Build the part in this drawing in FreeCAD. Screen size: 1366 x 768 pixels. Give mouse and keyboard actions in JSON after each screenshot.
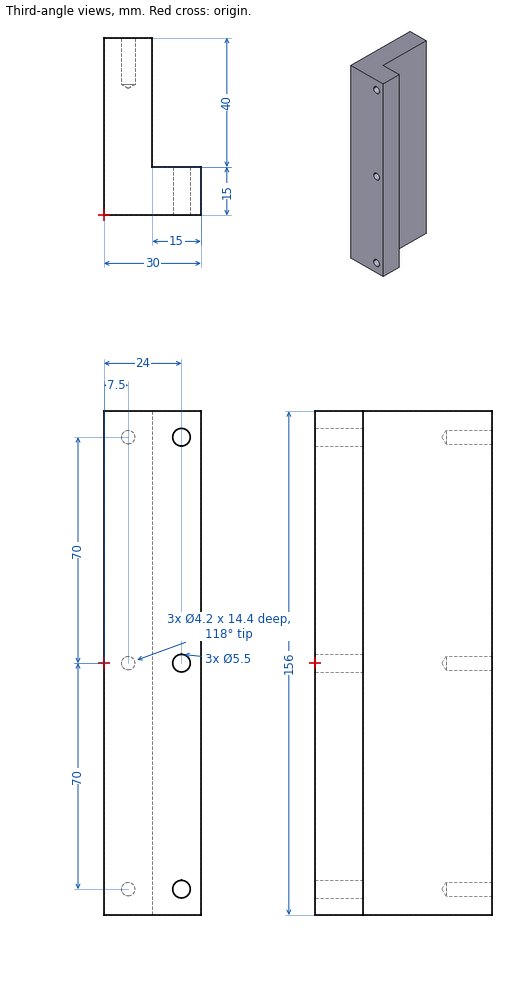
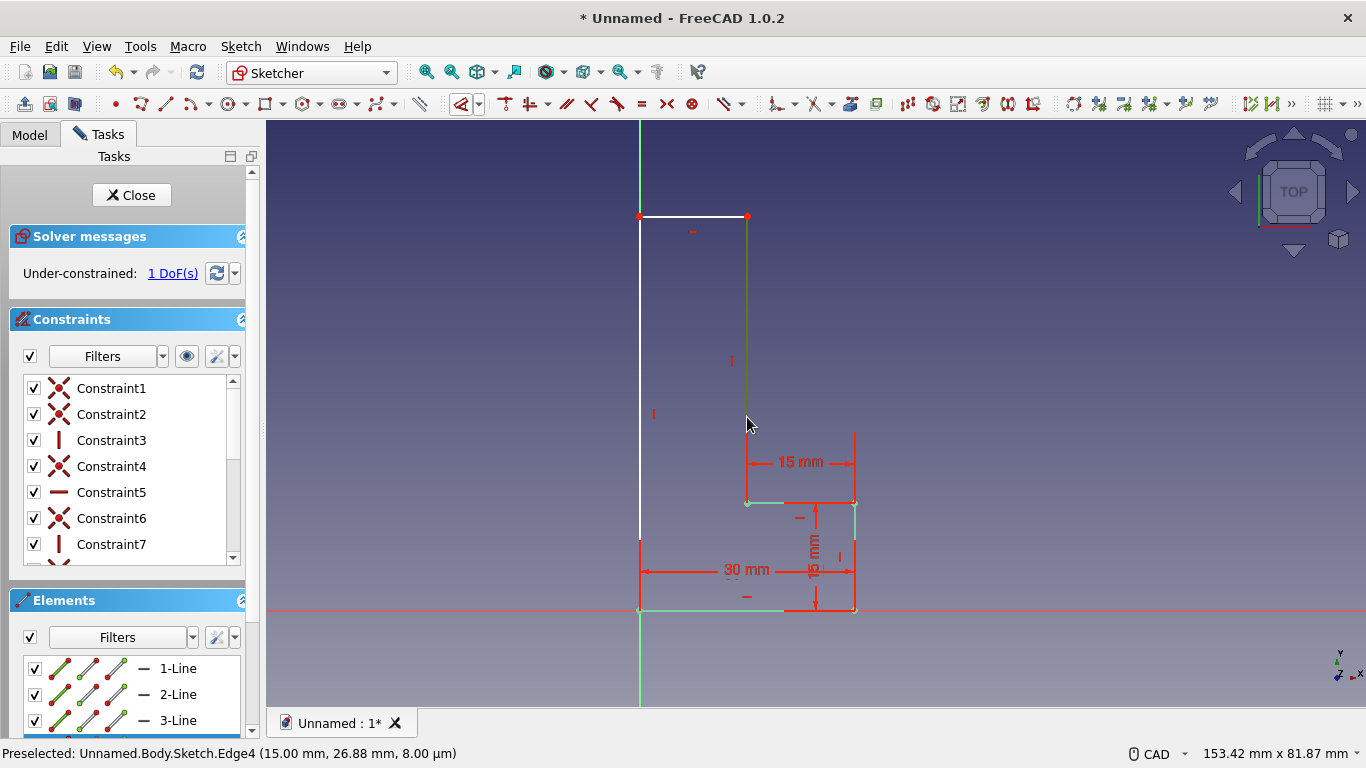
{"action": "key", "text": "i"}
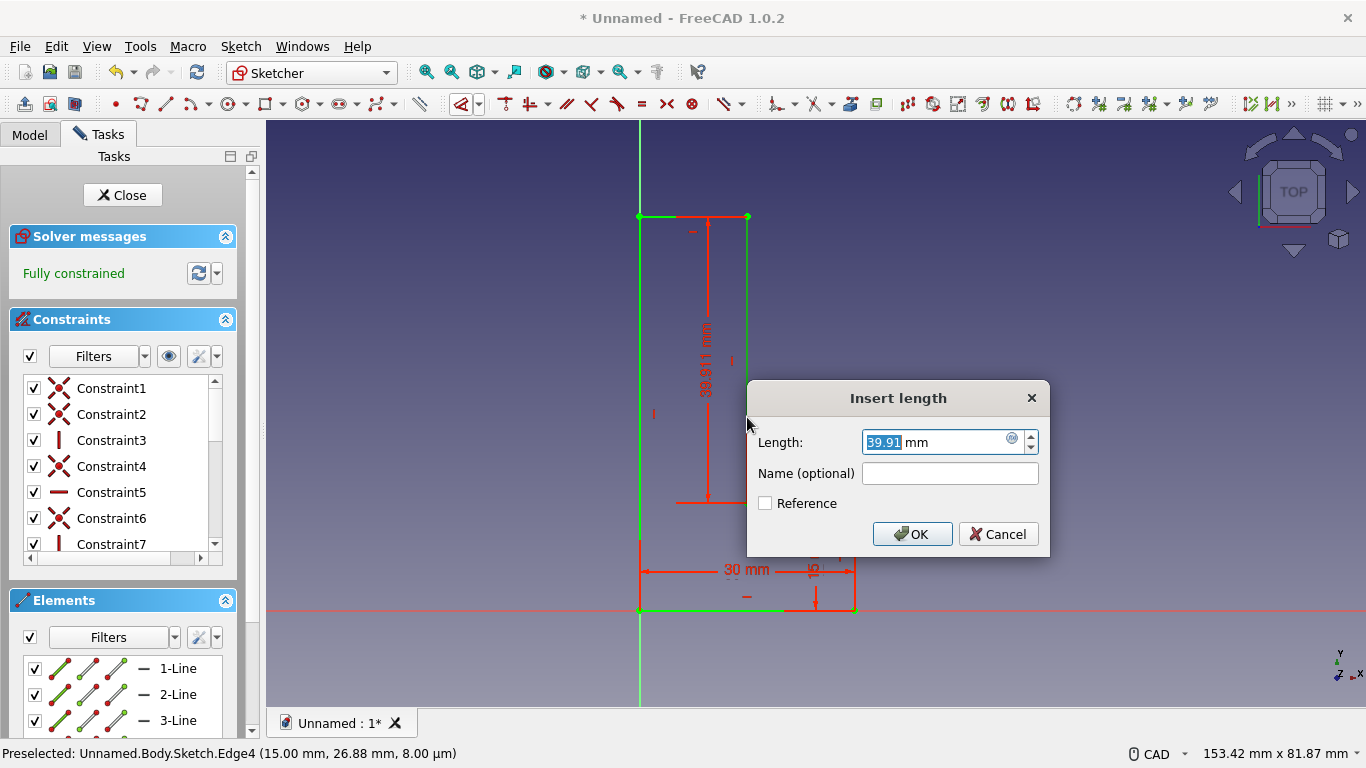
{"action": "type", "text": "40"}
{"action": "key", "text": "Return"}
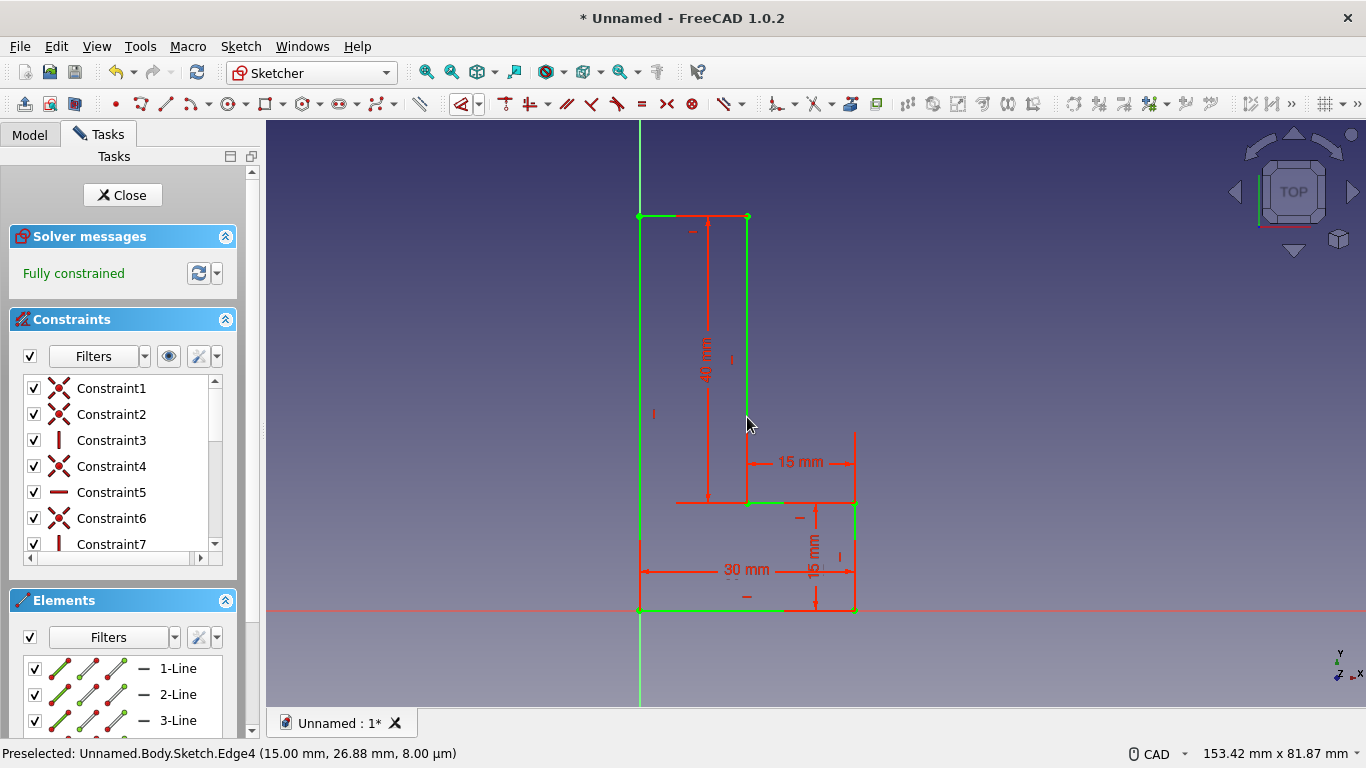
{"action": "left_click", "coordinate": [123, 195]}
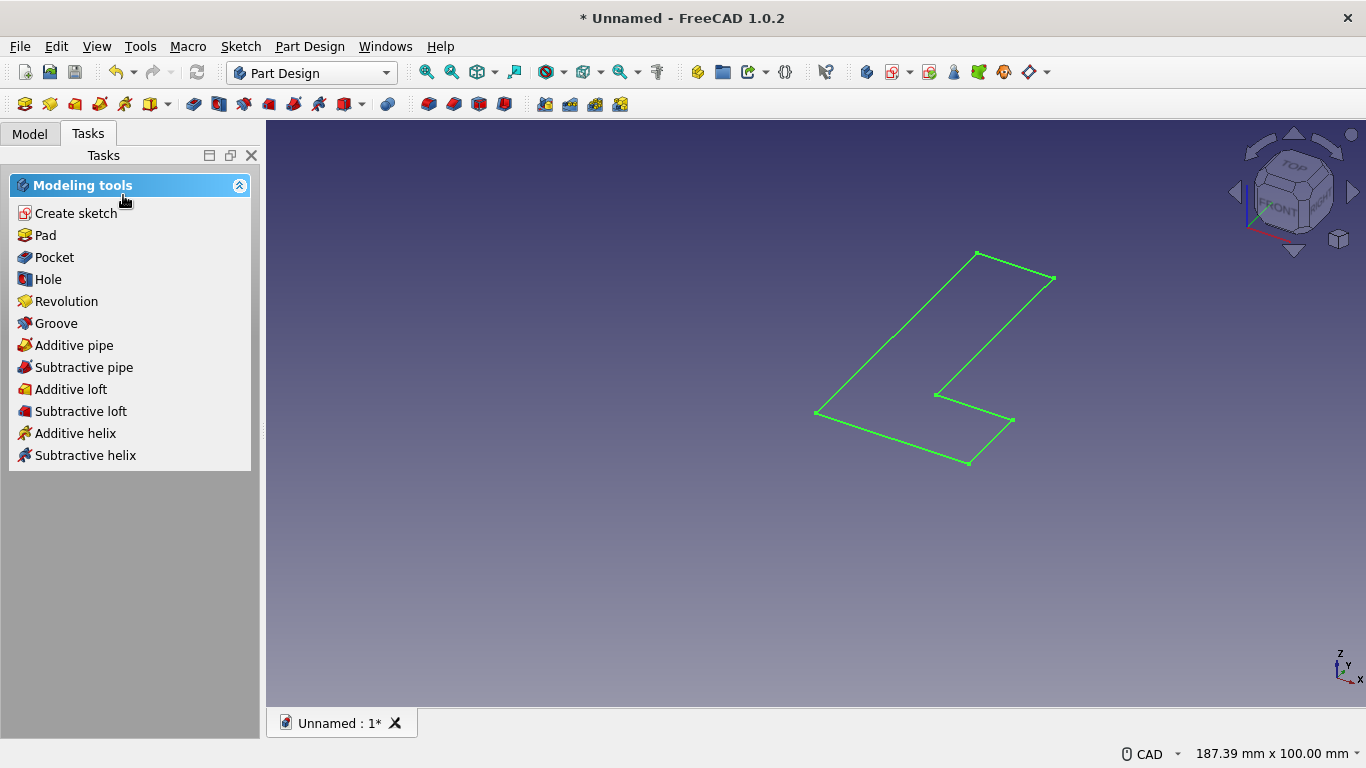
{"action": "left_click", "coordinate": [25, 104]}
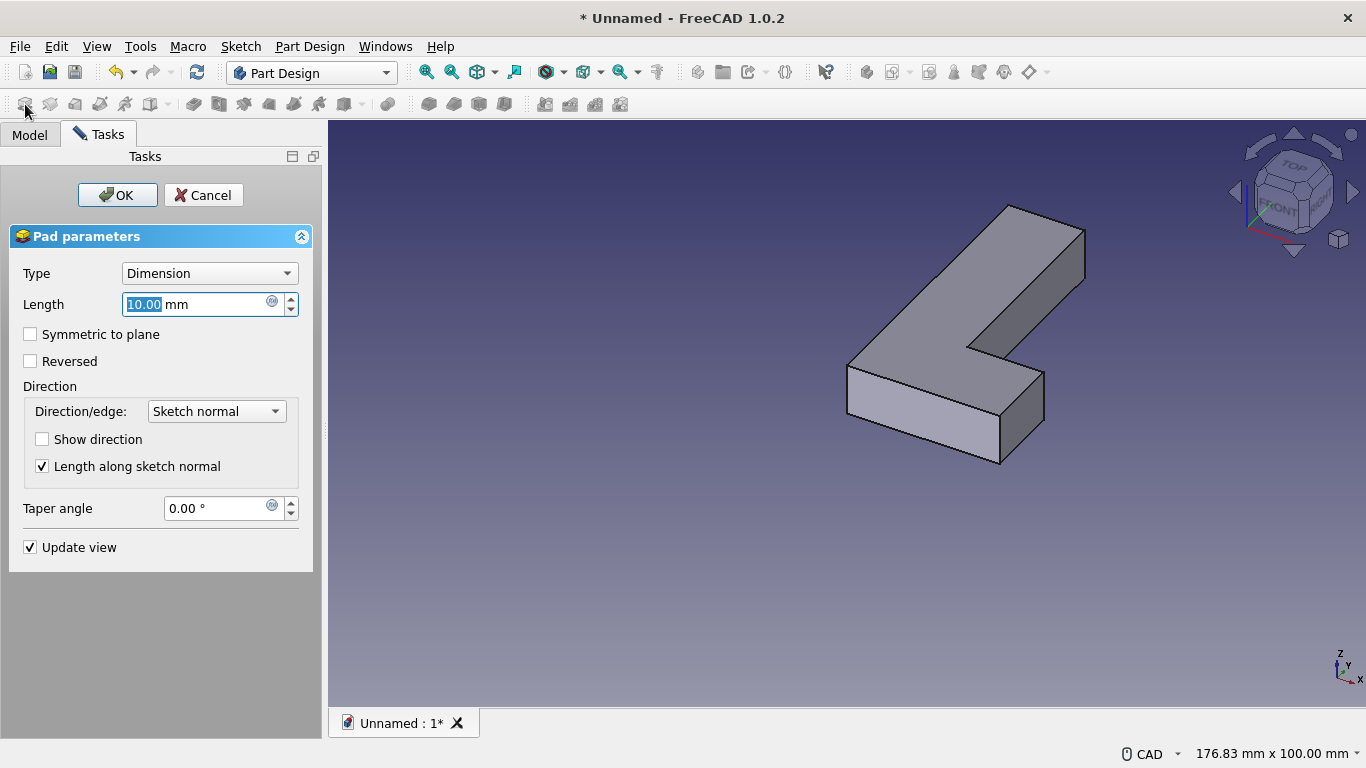
{"action": "type", "text": "156"}
{"action": "key", "text": "Tab"}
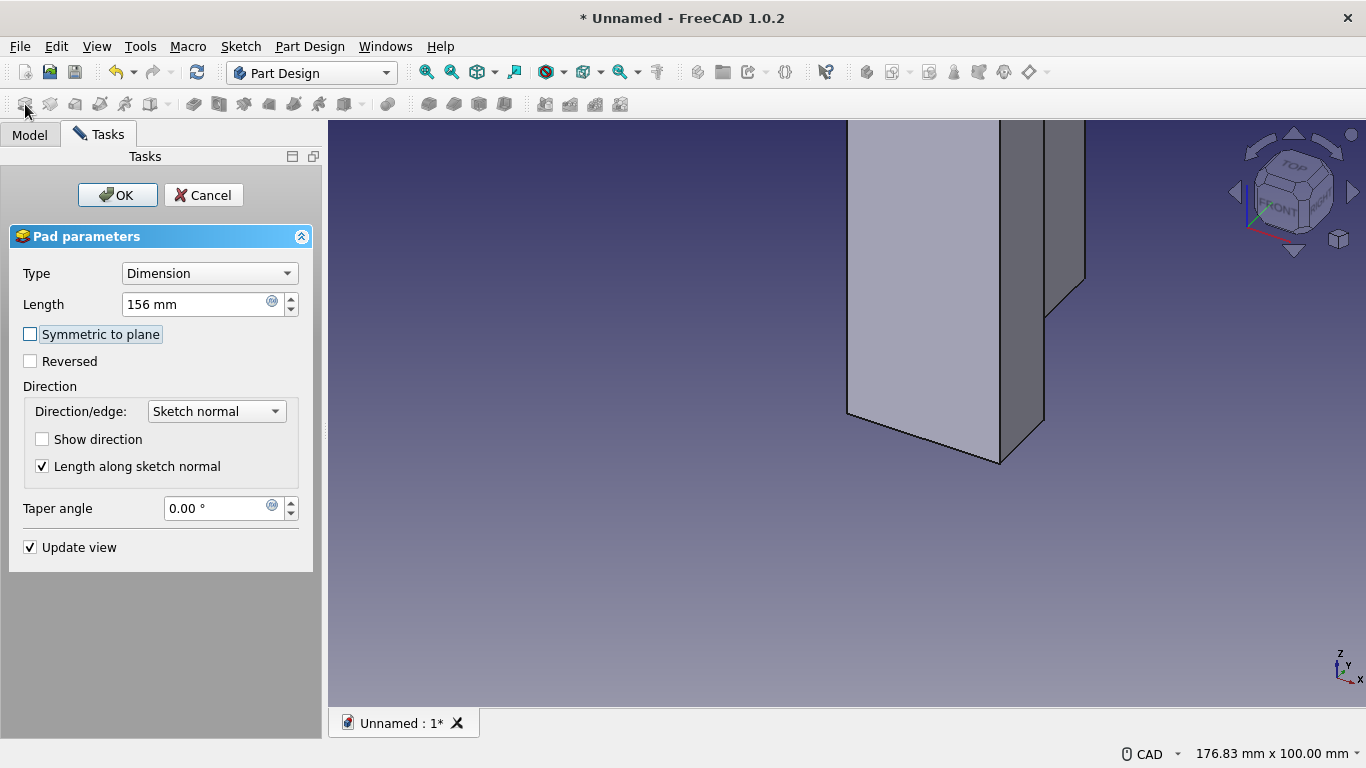
{"action": "left_click", "coordinate": [31, 334]}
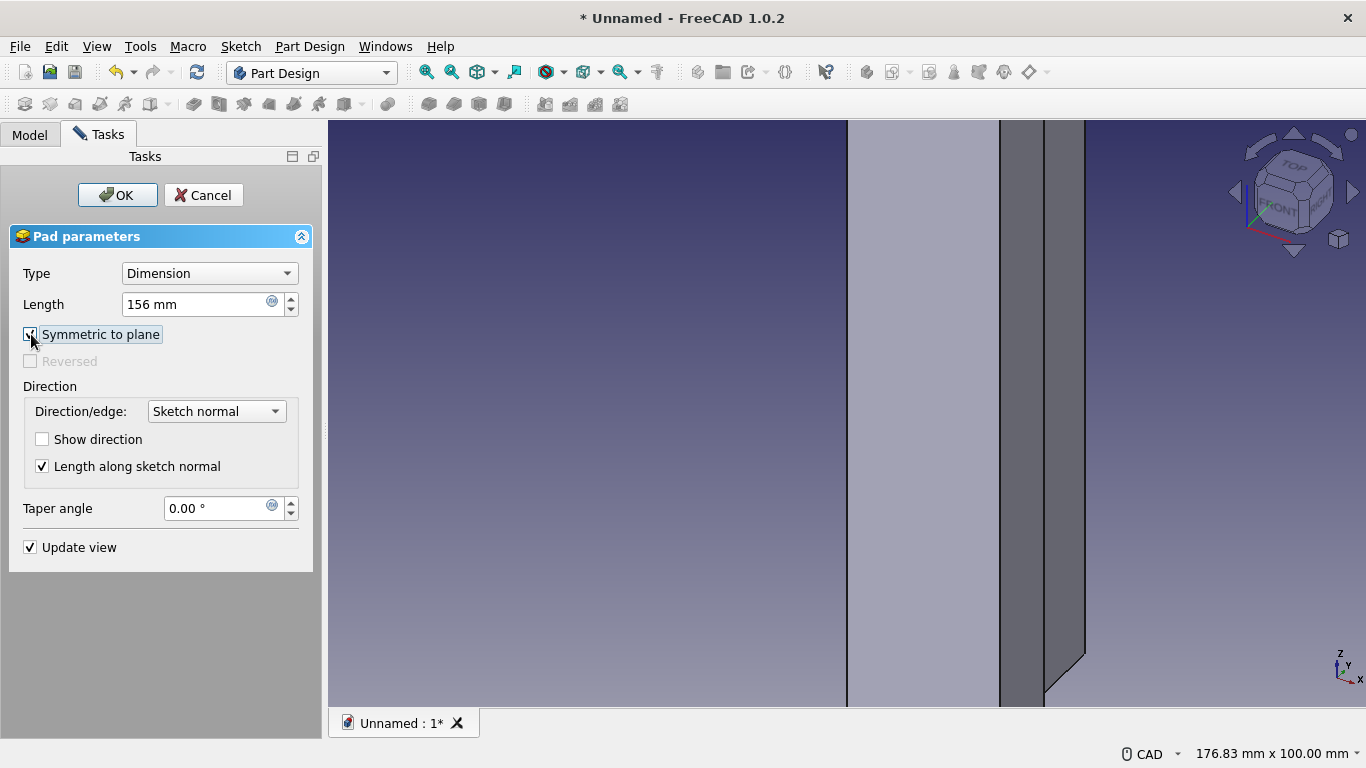
{"action": "left_click", "coordinate": [118, 195]}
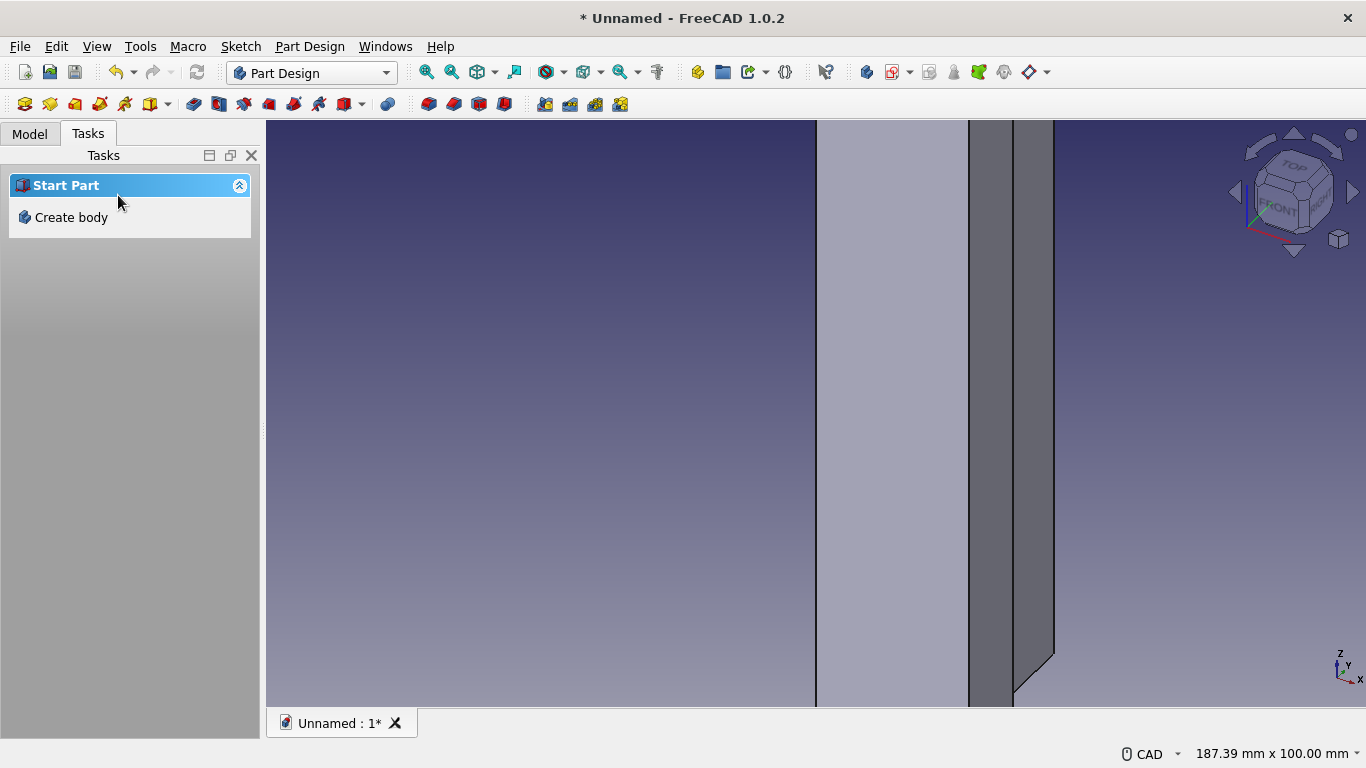
{"action": "key", "text": "v f"}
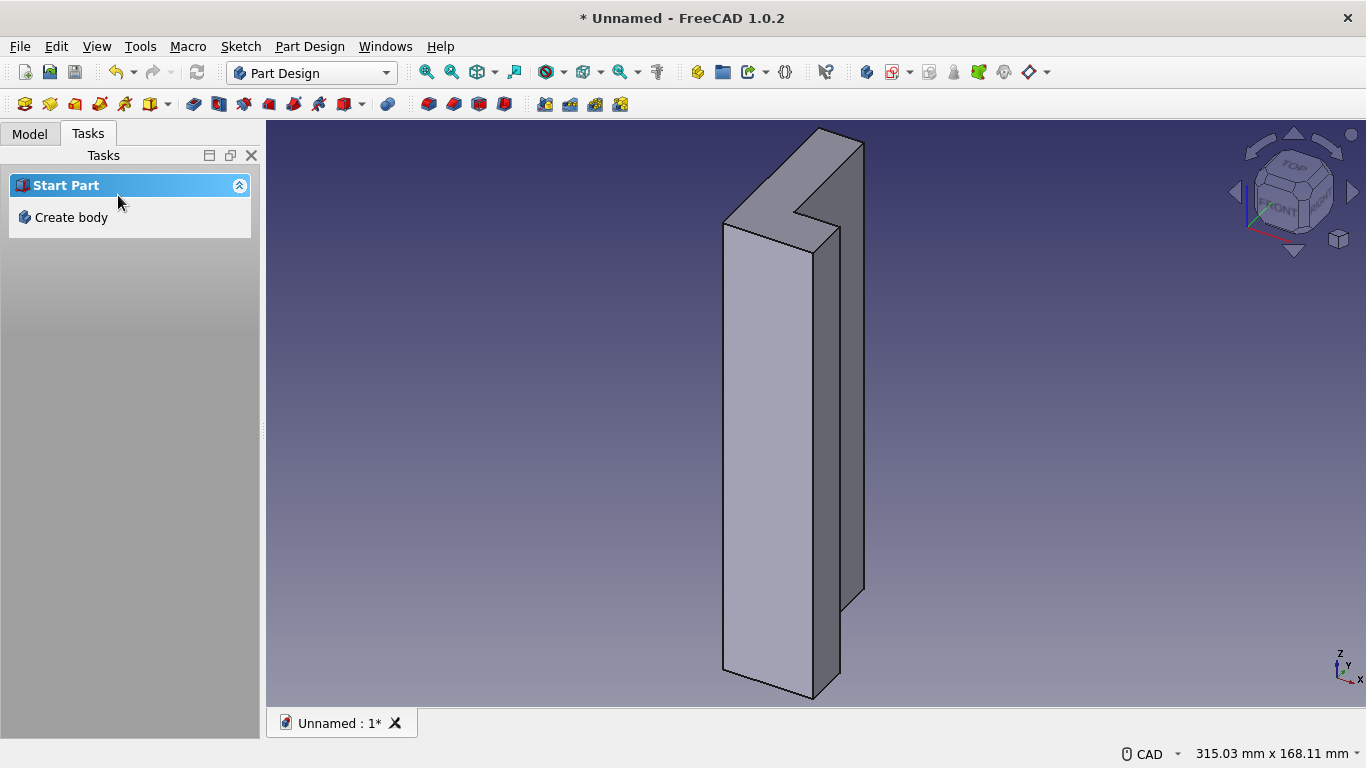
{"action": "key", "text": "4"}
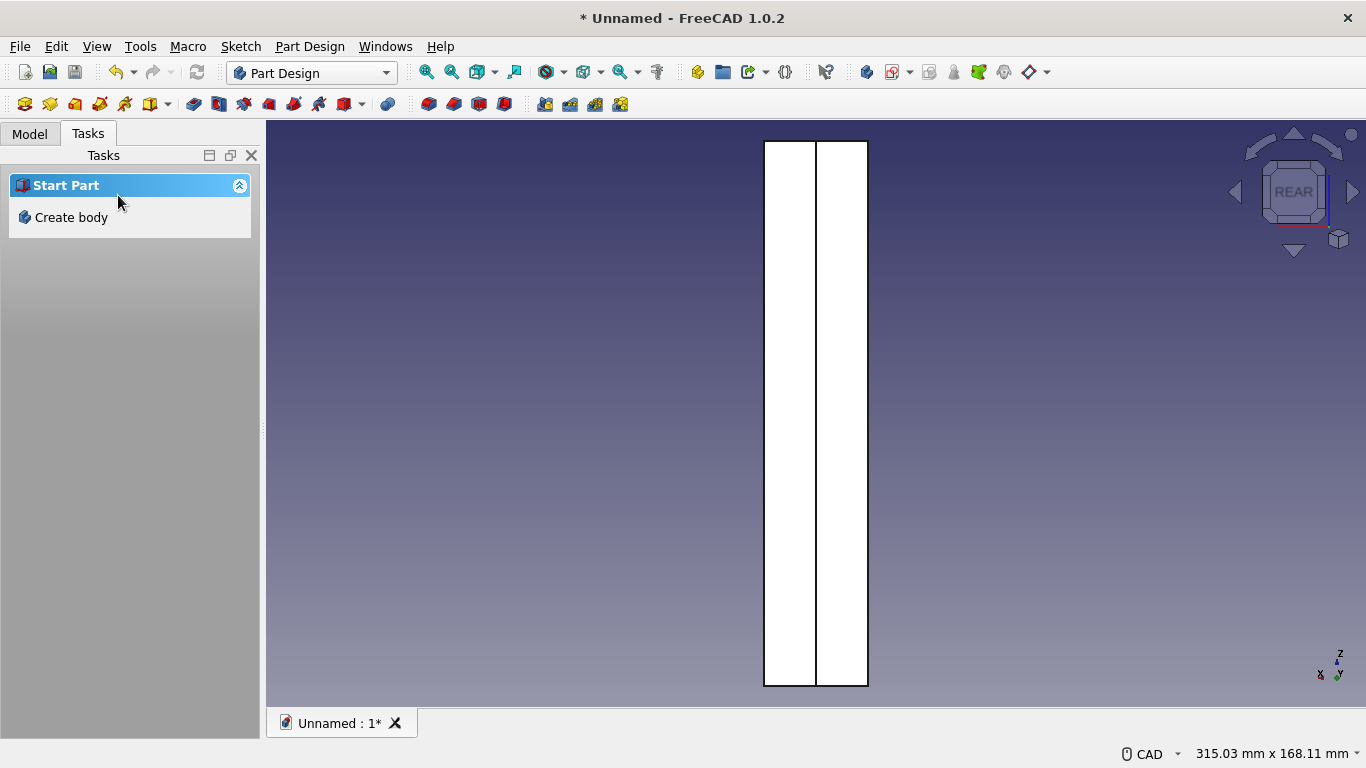
{"action": "left_click", "coordinate": [842, 179]}